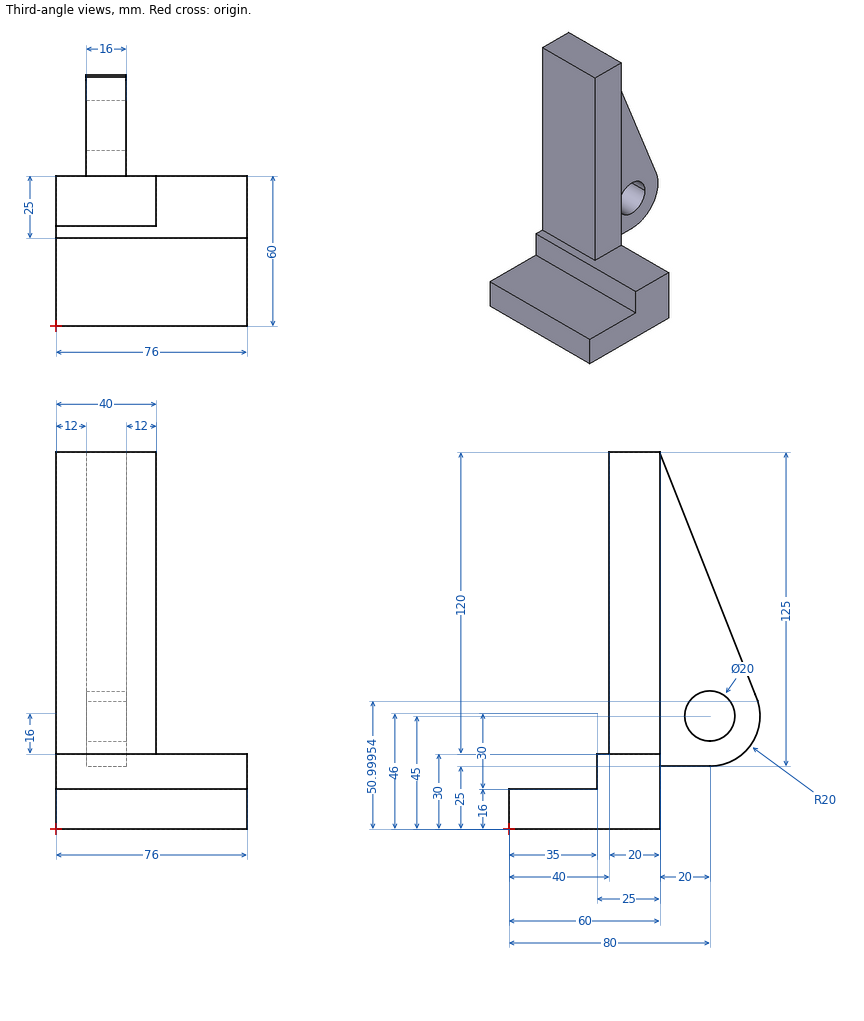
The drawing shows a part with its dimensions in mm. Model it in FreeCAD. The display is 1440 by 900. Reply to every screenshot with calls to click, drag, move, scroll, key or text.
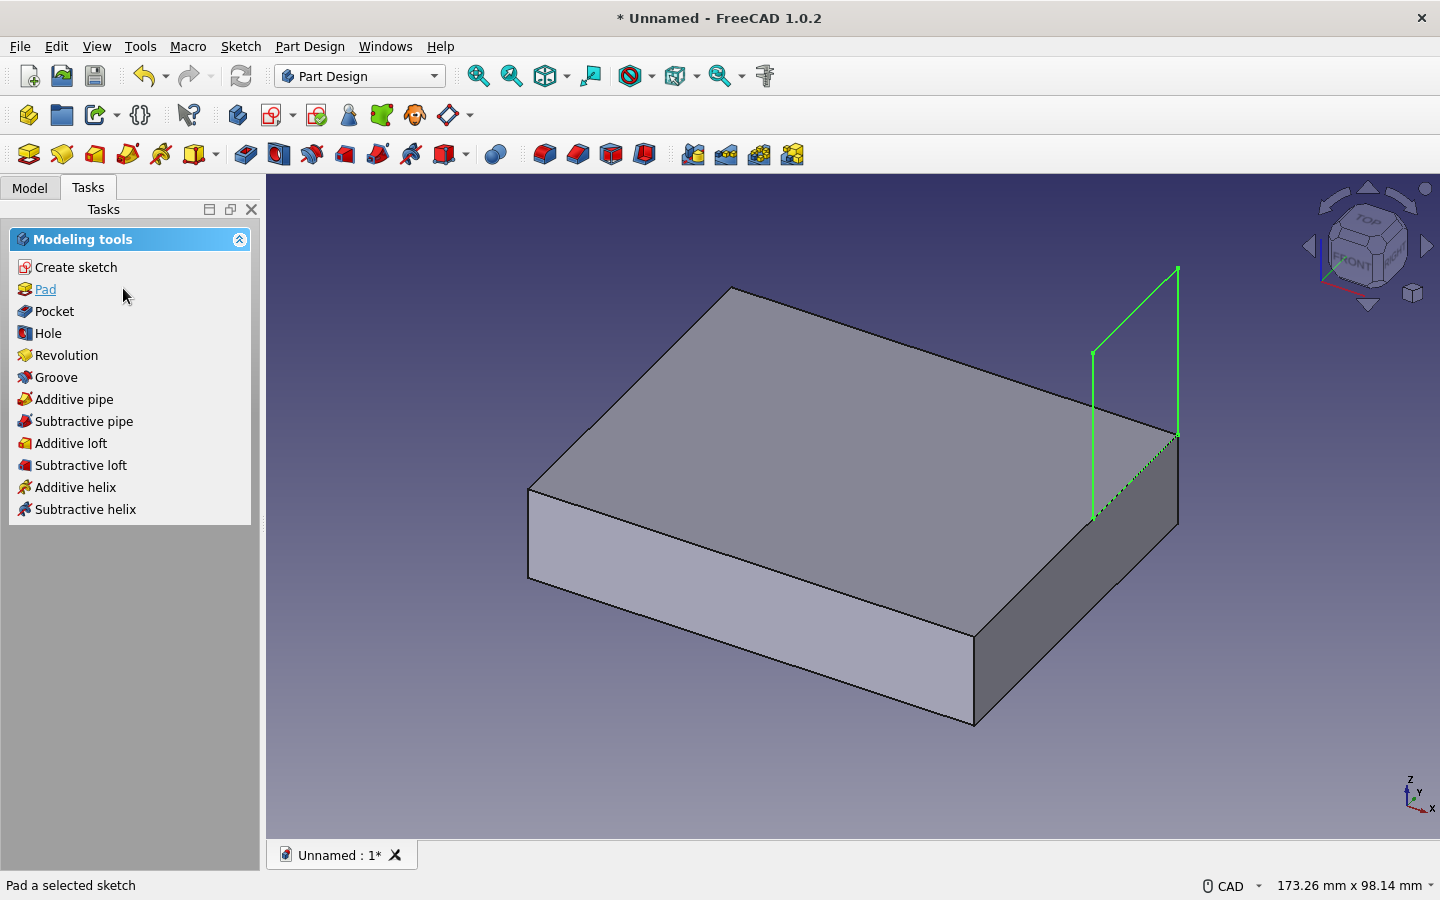
click(29, 154)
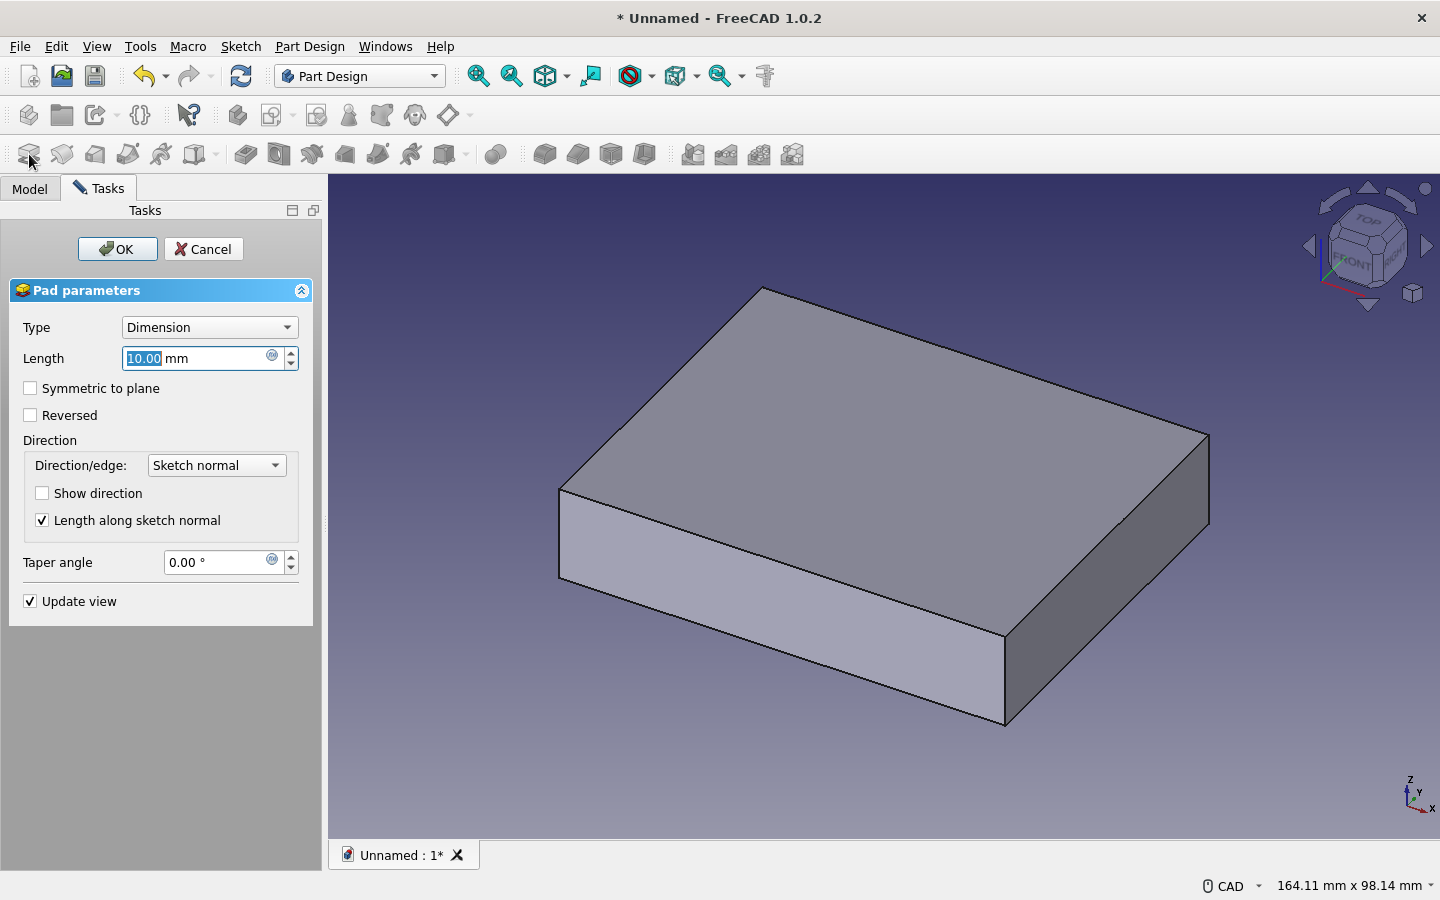
text(76)
key(Tab)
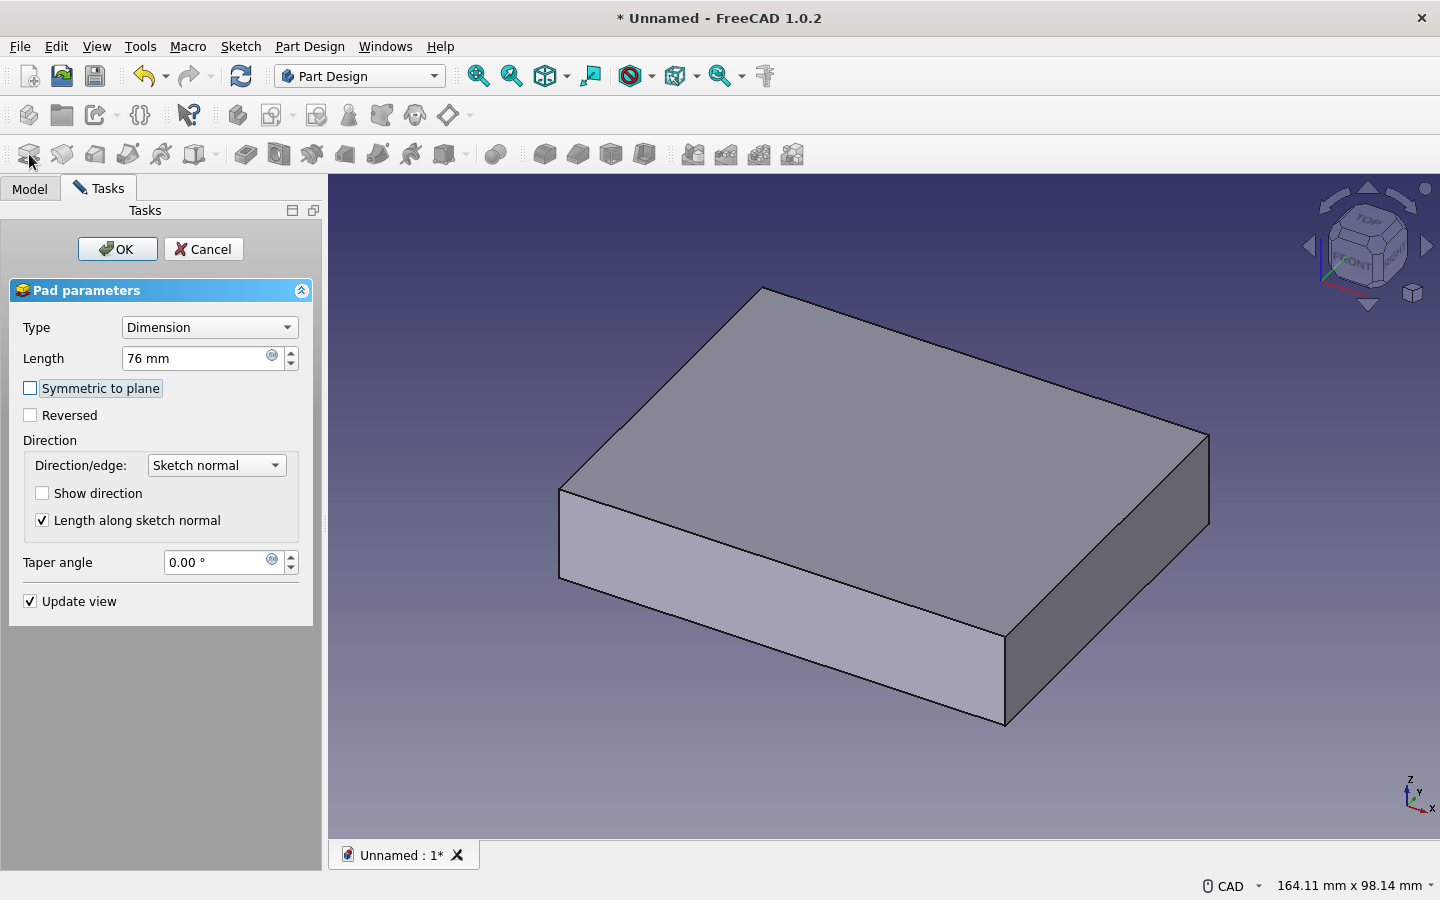
click(31, 415)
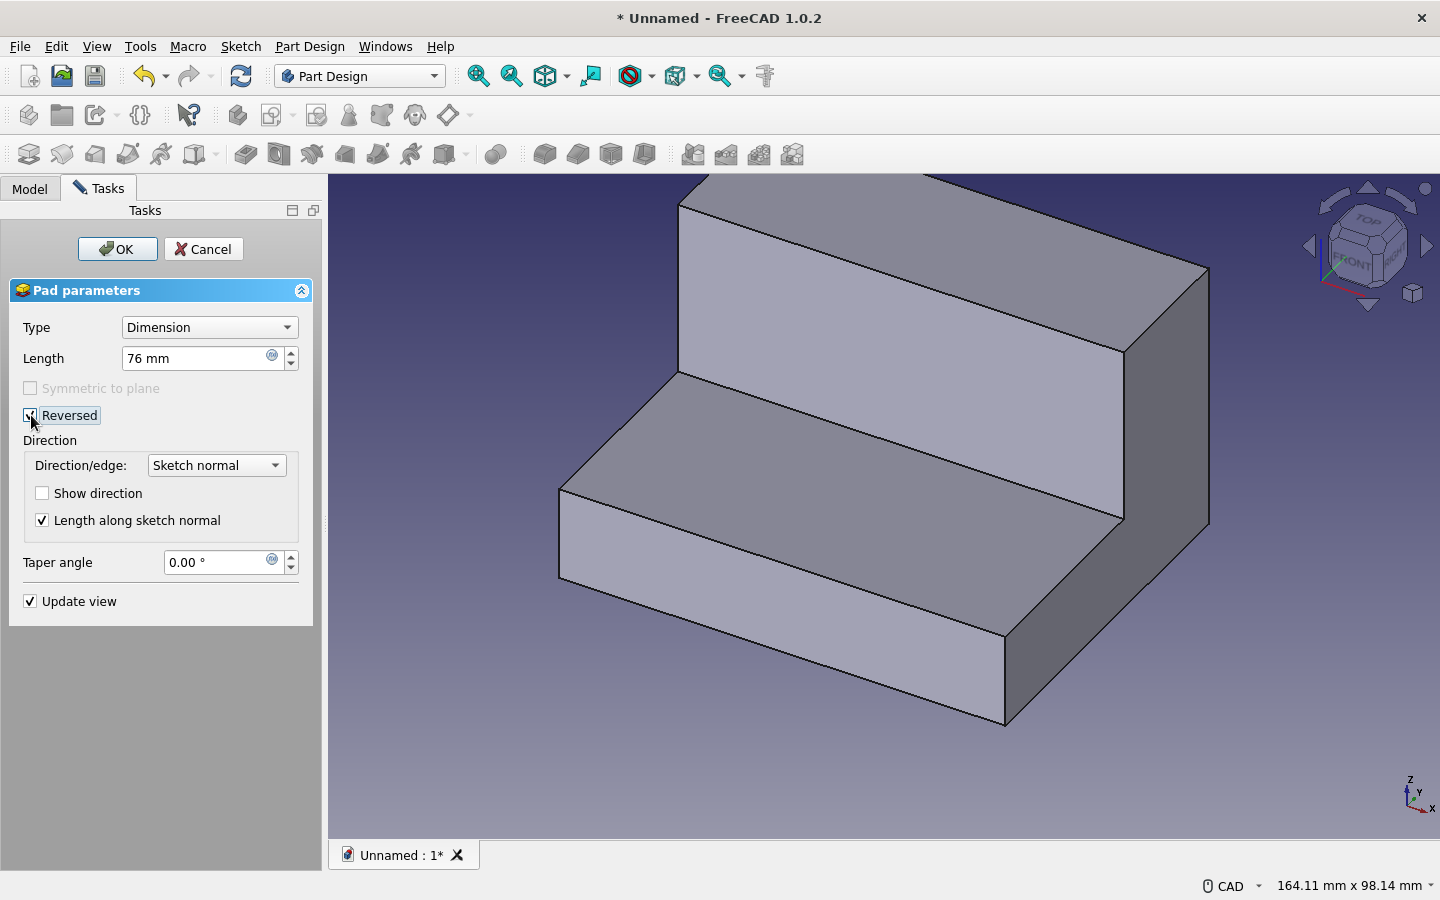
click(118, 249)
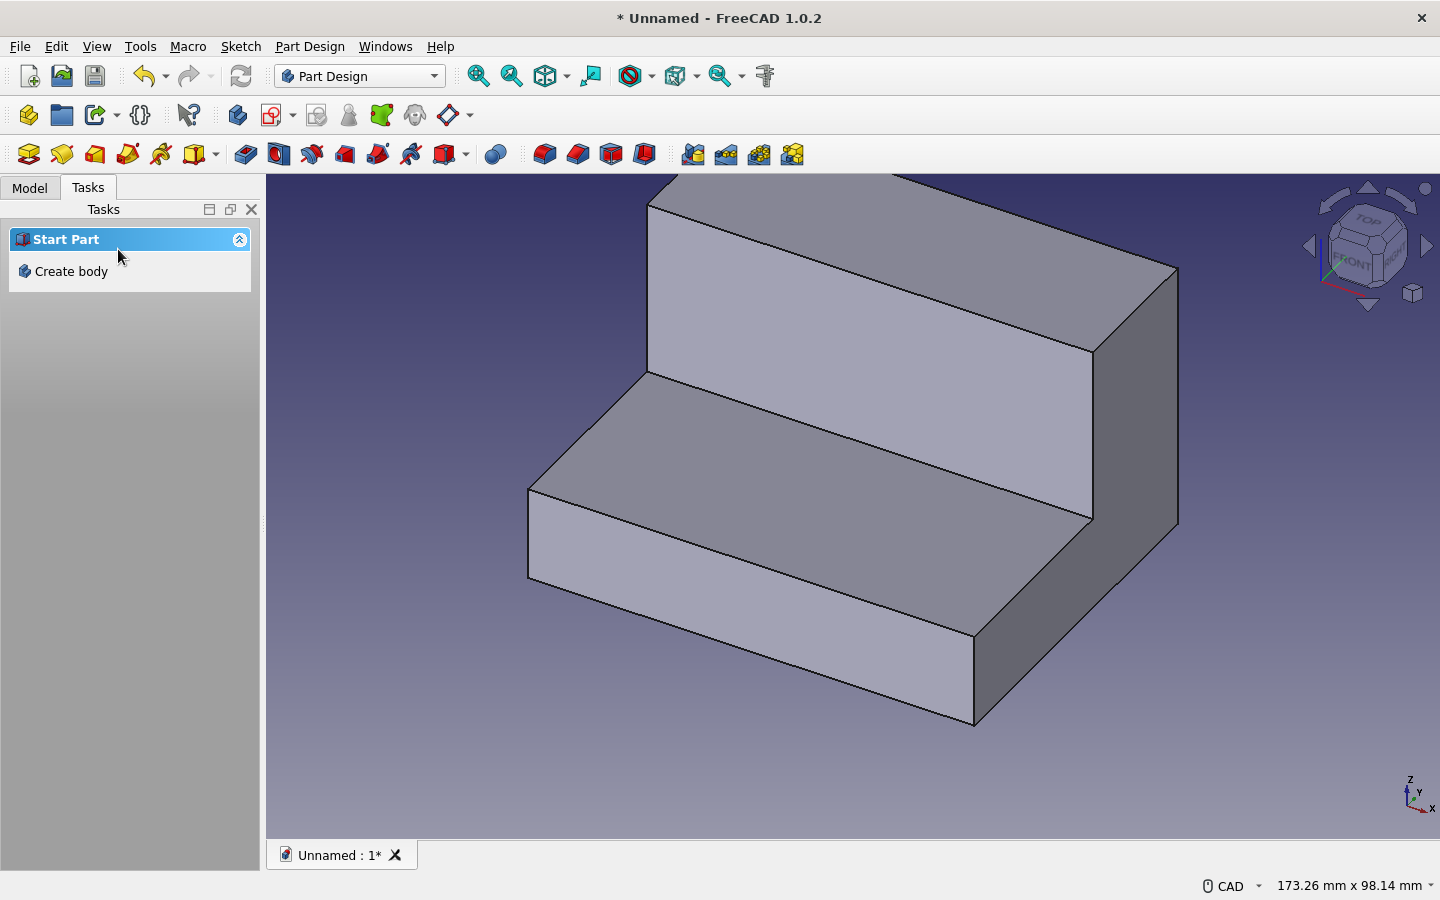
click(479, 76)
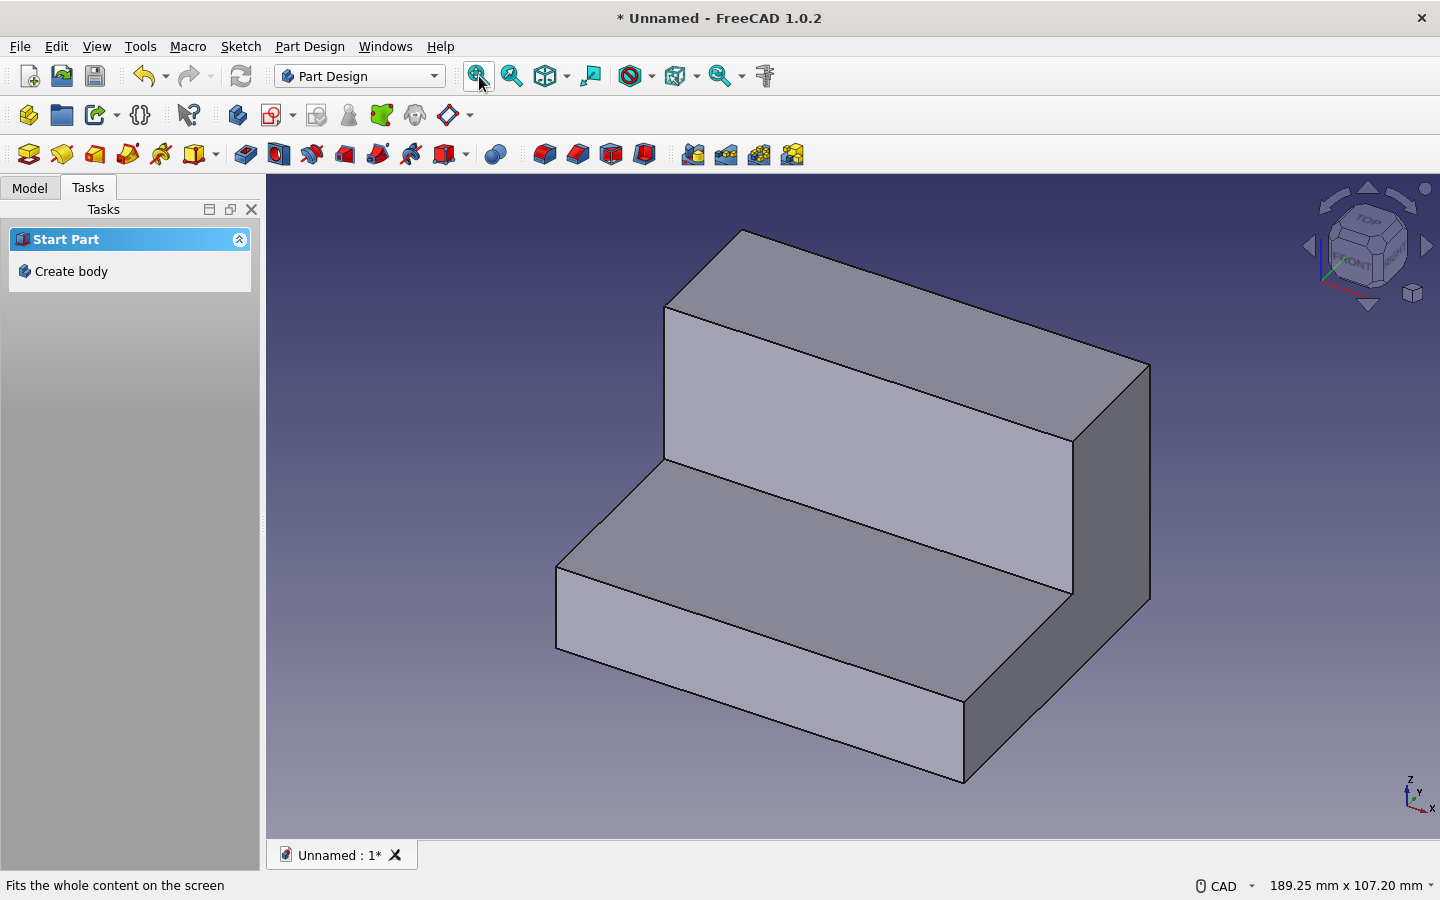
click(1024, 373)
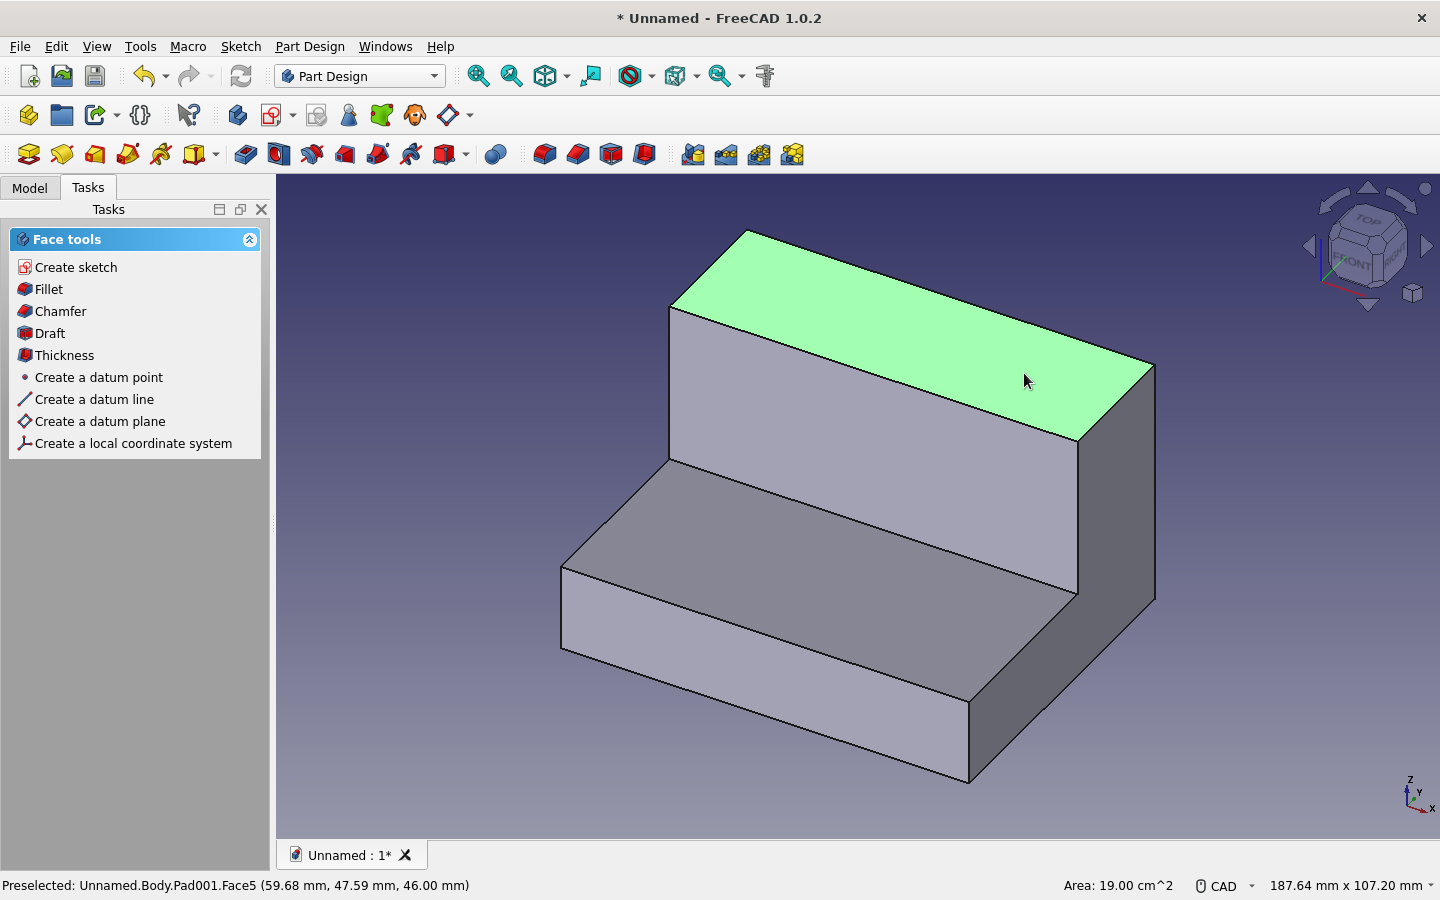
click(270, 116)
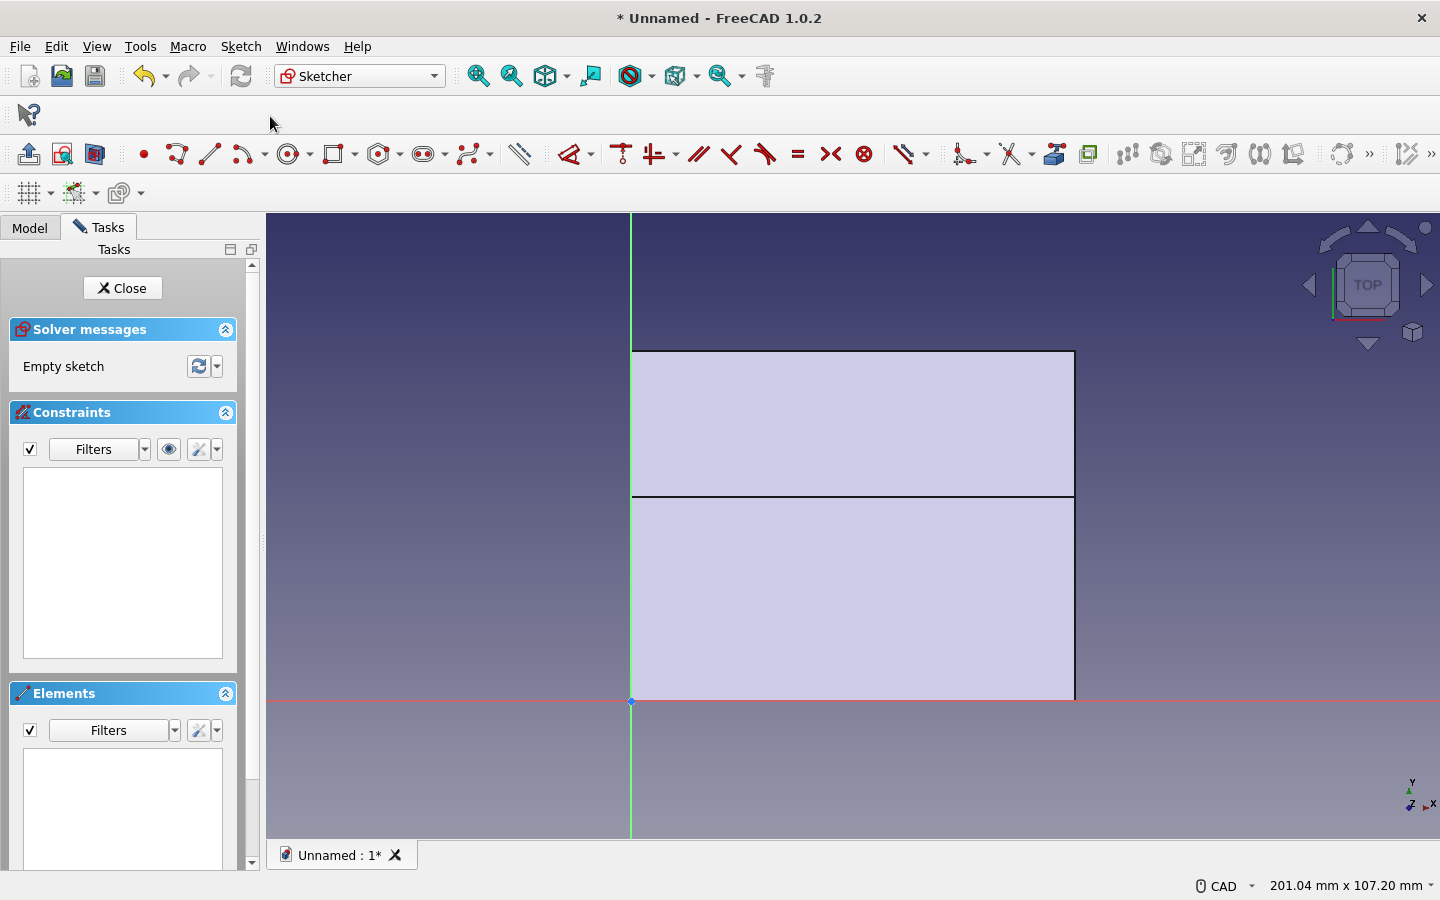
key(g)
key(r)